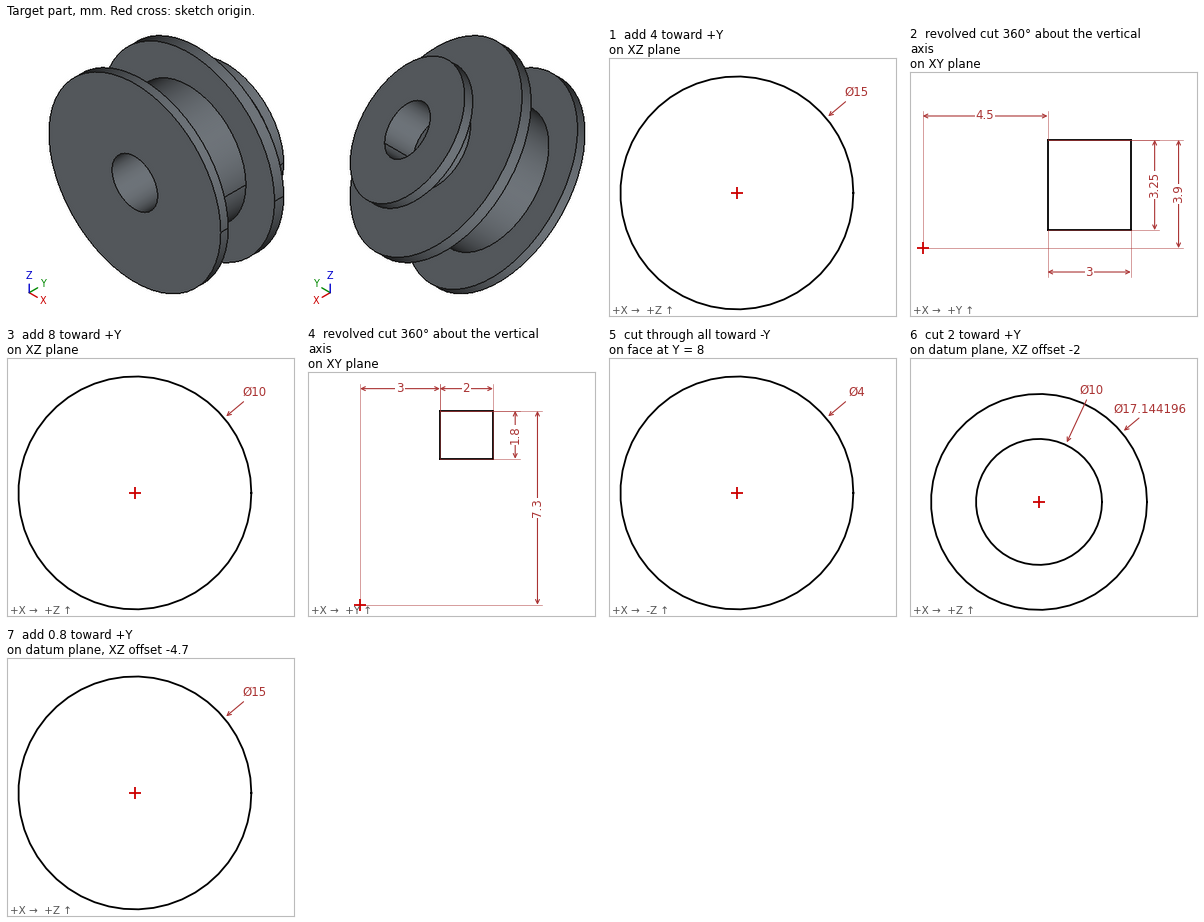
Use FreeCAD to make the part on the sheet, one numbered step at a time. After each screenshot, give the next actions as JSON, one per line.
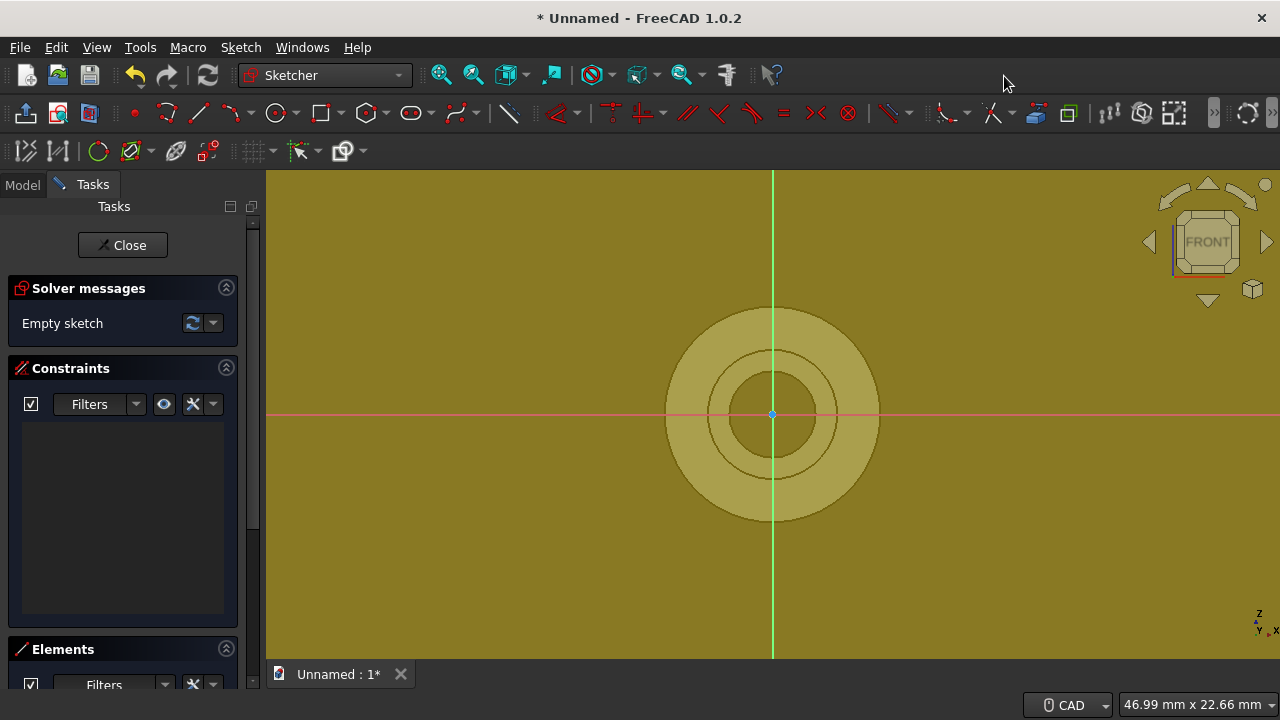
{"action": "key", "text": "g c"}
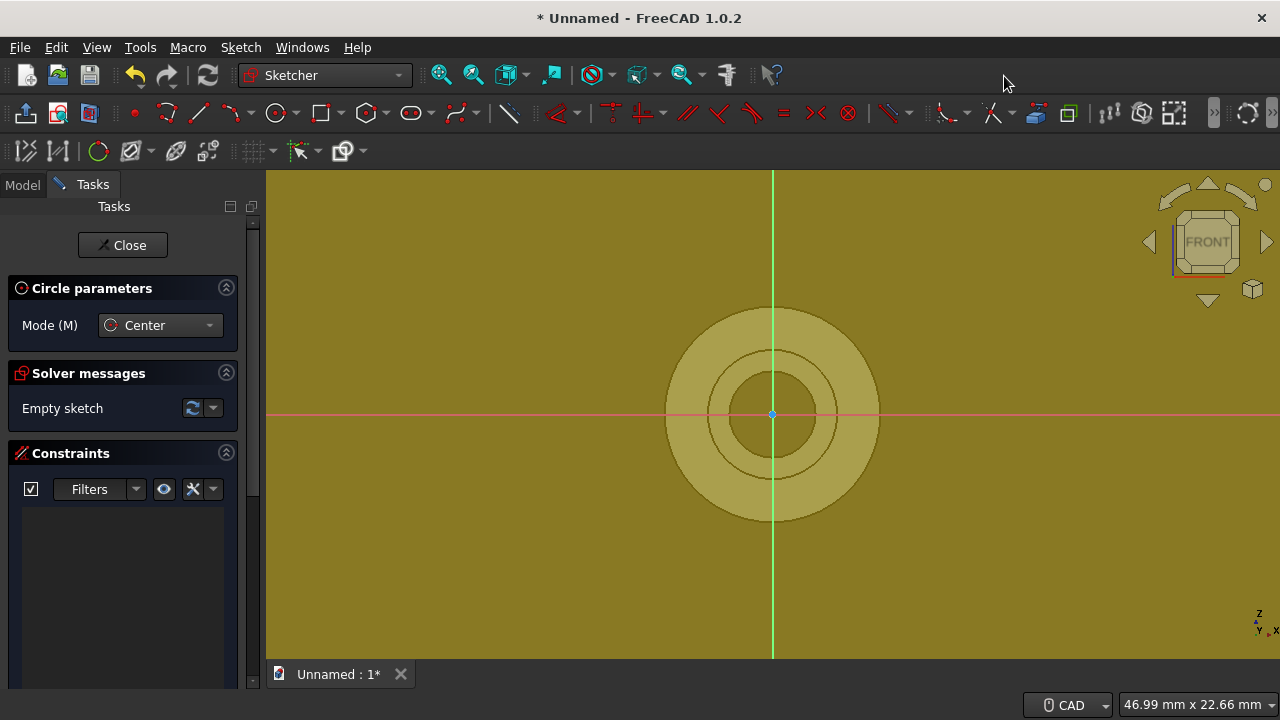
{"action": "left_click", "coordinate": [773, 415]}
{"action": "left_click", "coordinate": [887, 300]}
{"action": "key", "text": "Escape"}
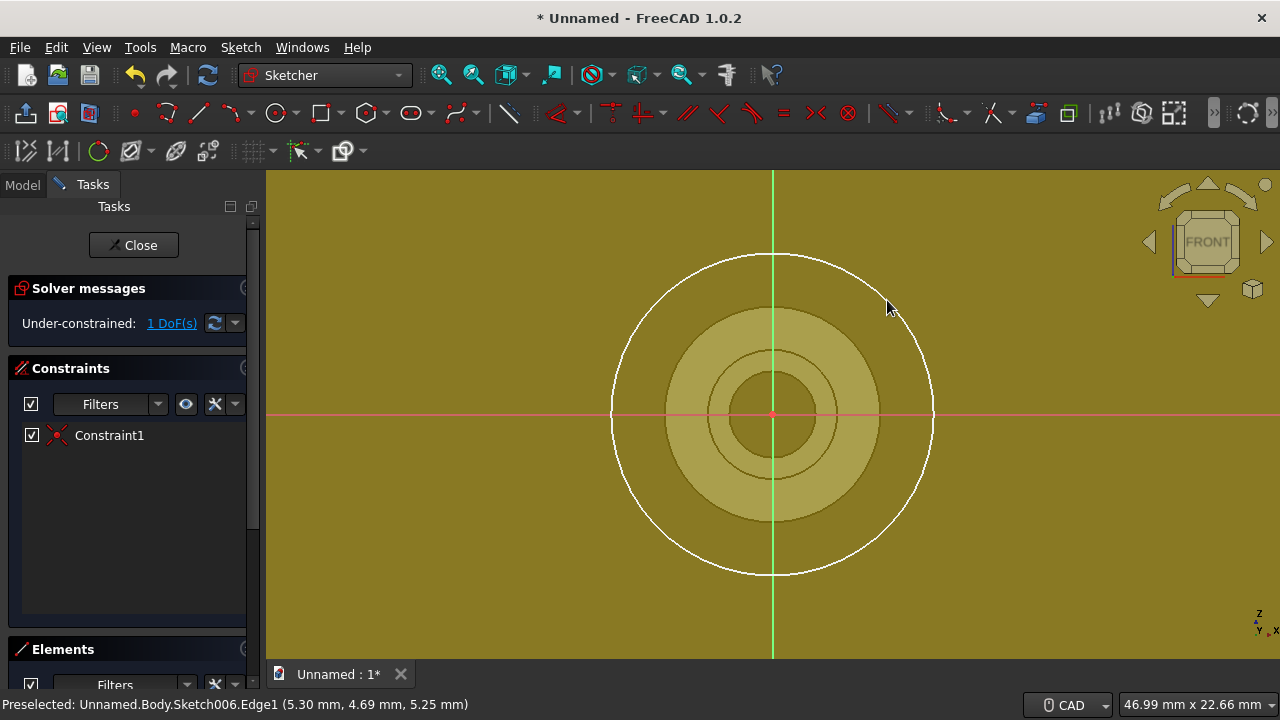
{"action": "key", "text": "d"}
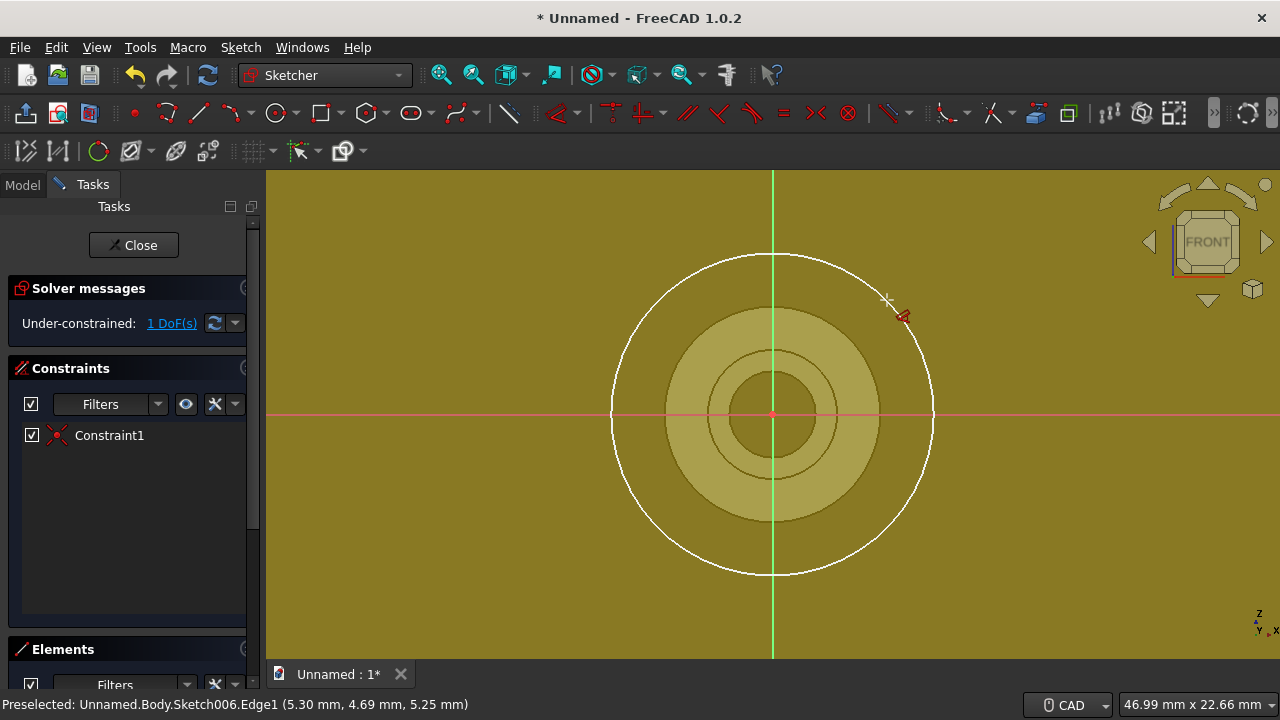
{"action": "left_click", "coordinate": [886, 300]}
{"action": "left_click", "coordinate": [909, 277]}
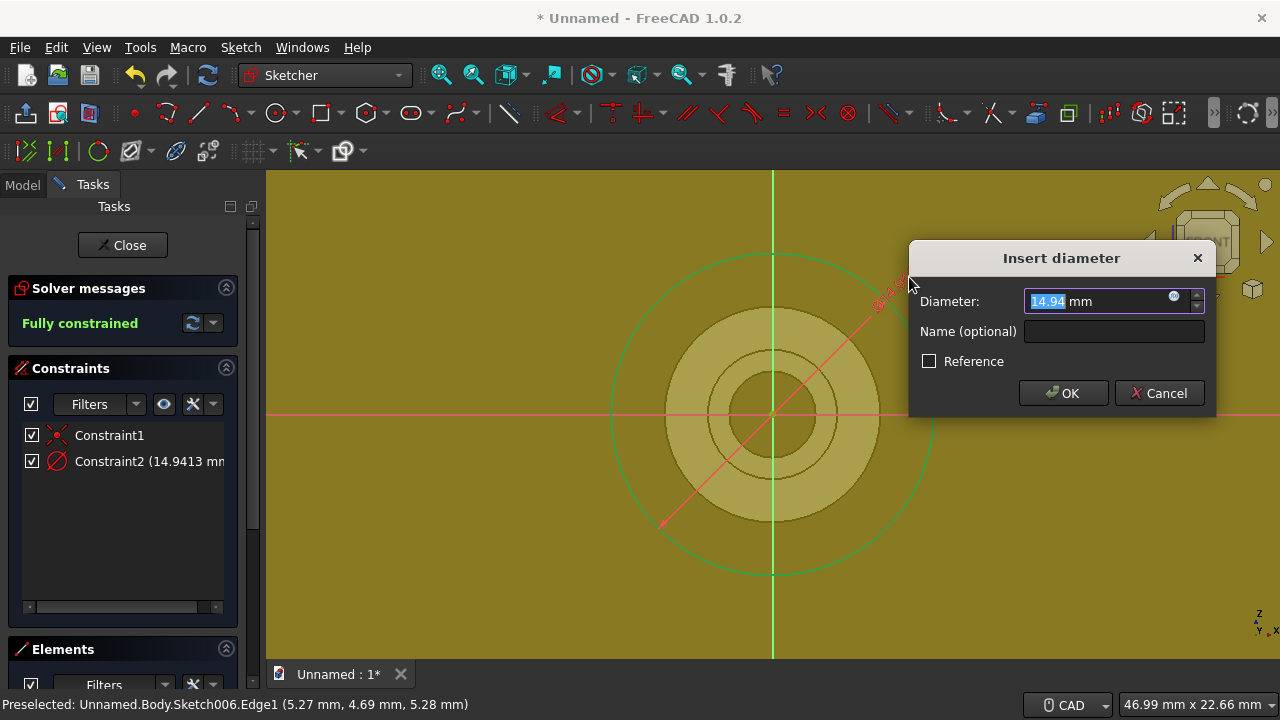
{"action": "type", "text": "15"}
{"action": "key", "text": "Return"}
{"action": "key", "text": "Escape"}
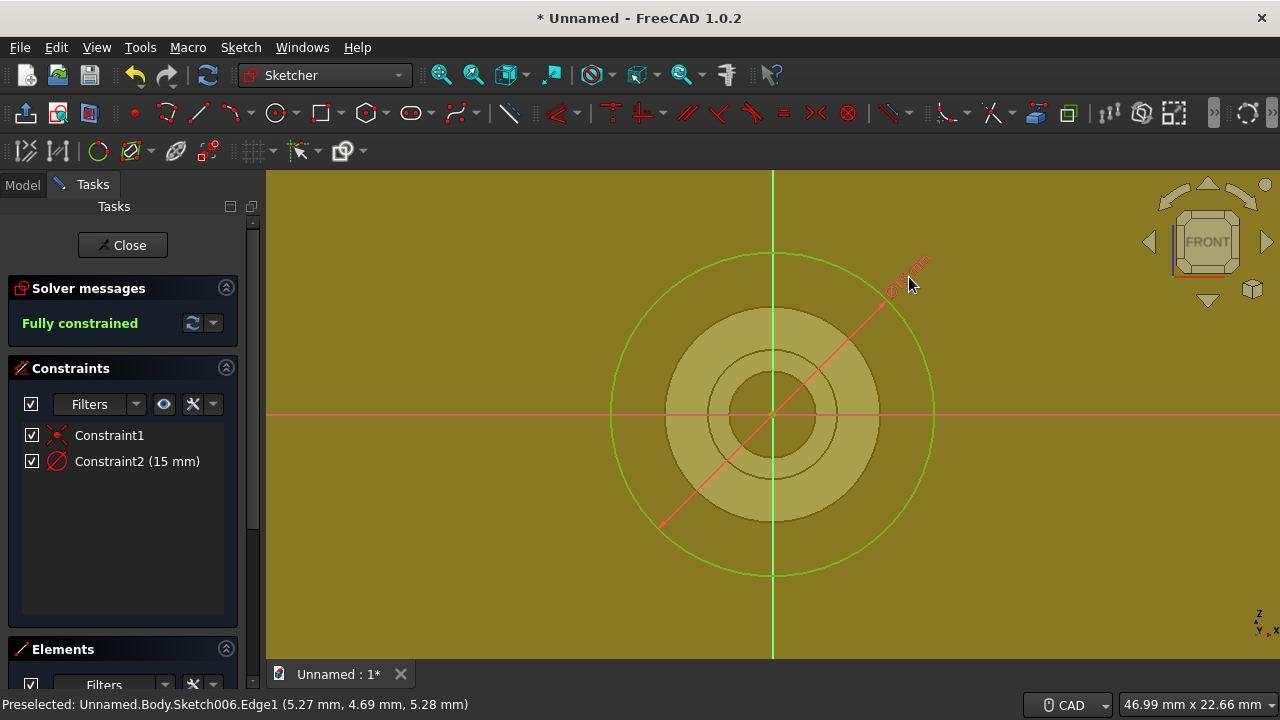
{"action": "left_click", "coordinate": [123, 245]}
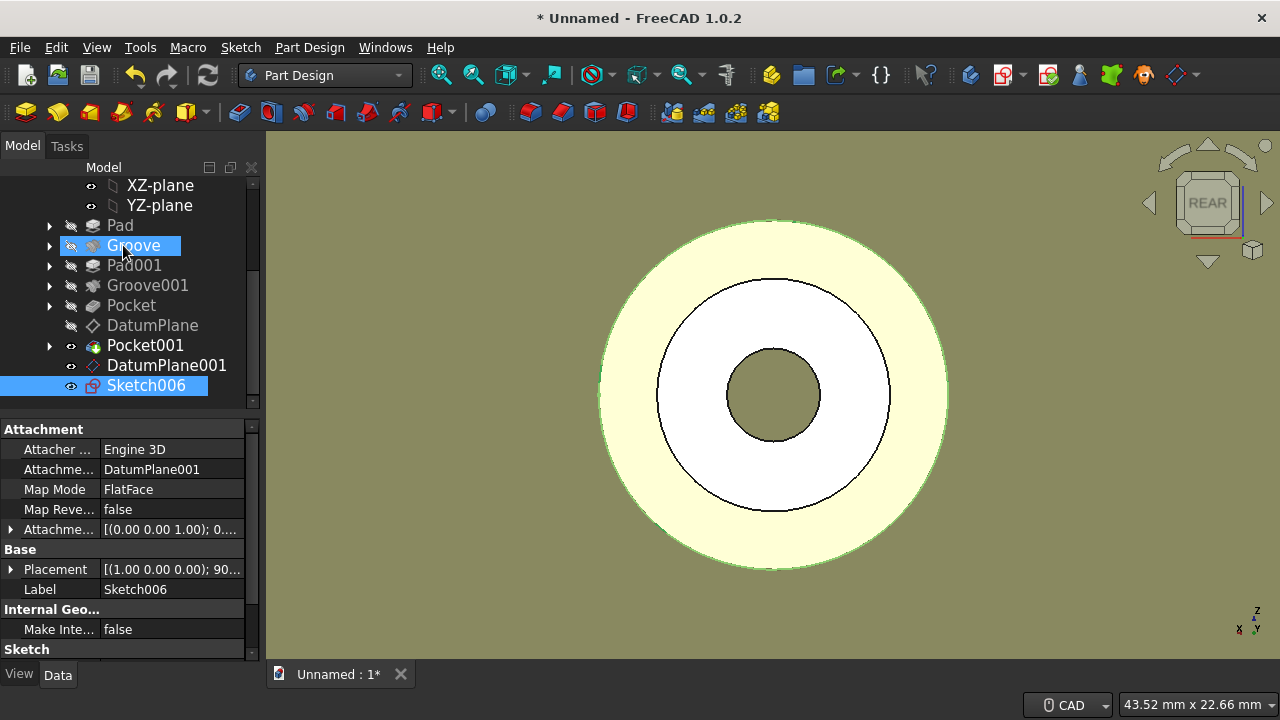
{"action": "left_click", "coordinate": [26, 112]}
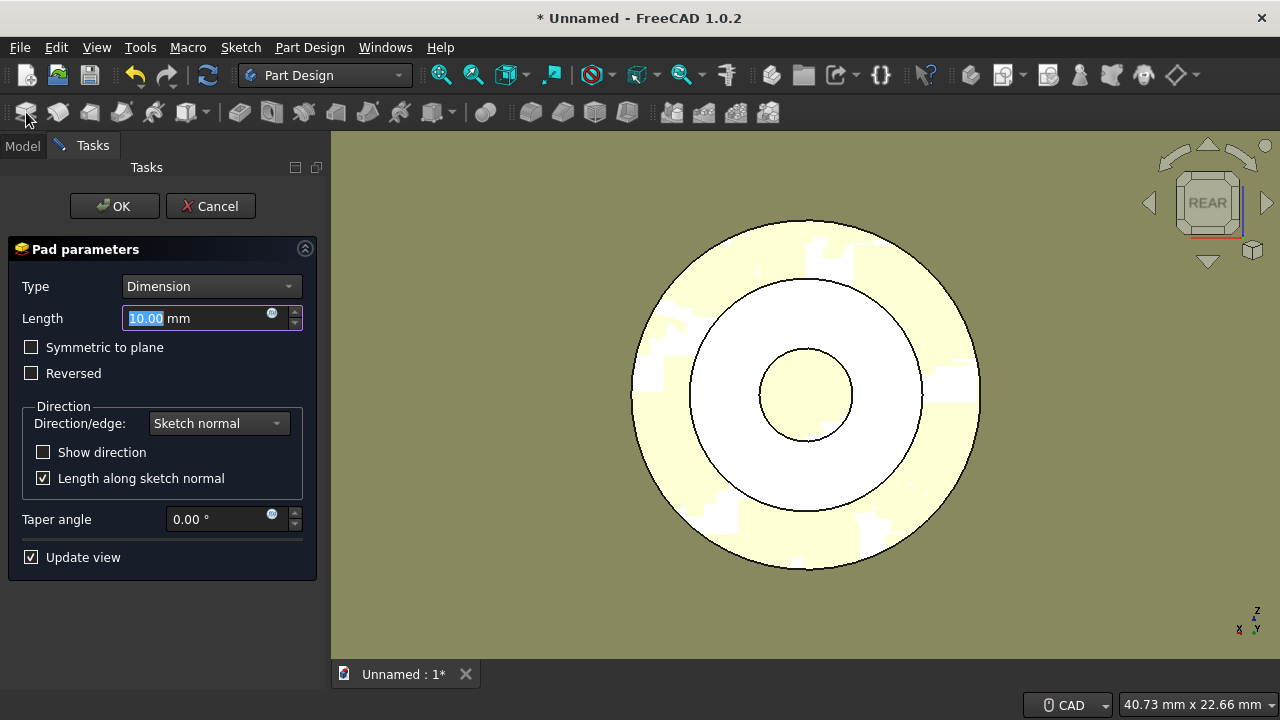
{"action": "type", "text": "0.8"}
{"action": "key", "text": "Tab"}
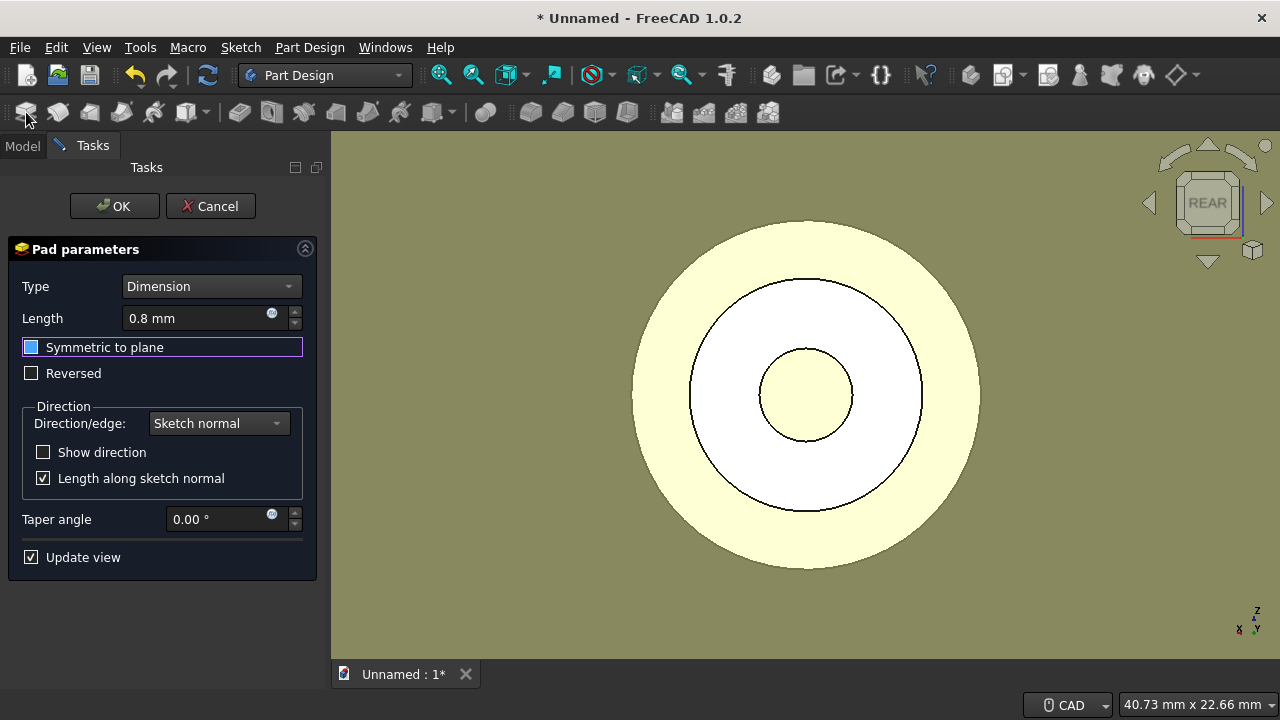
{"action": "left_click", "coordinate": [30, 373]}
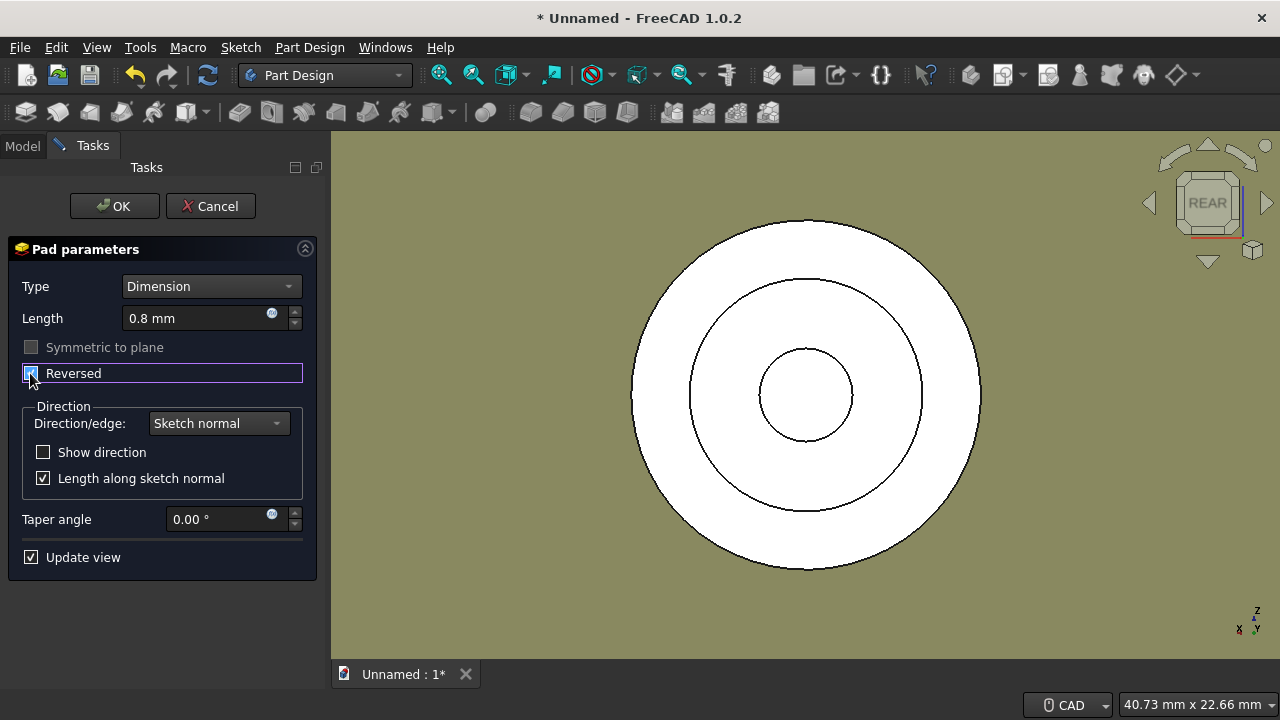
{"action": "left_click", "coordinate": [115, 206]}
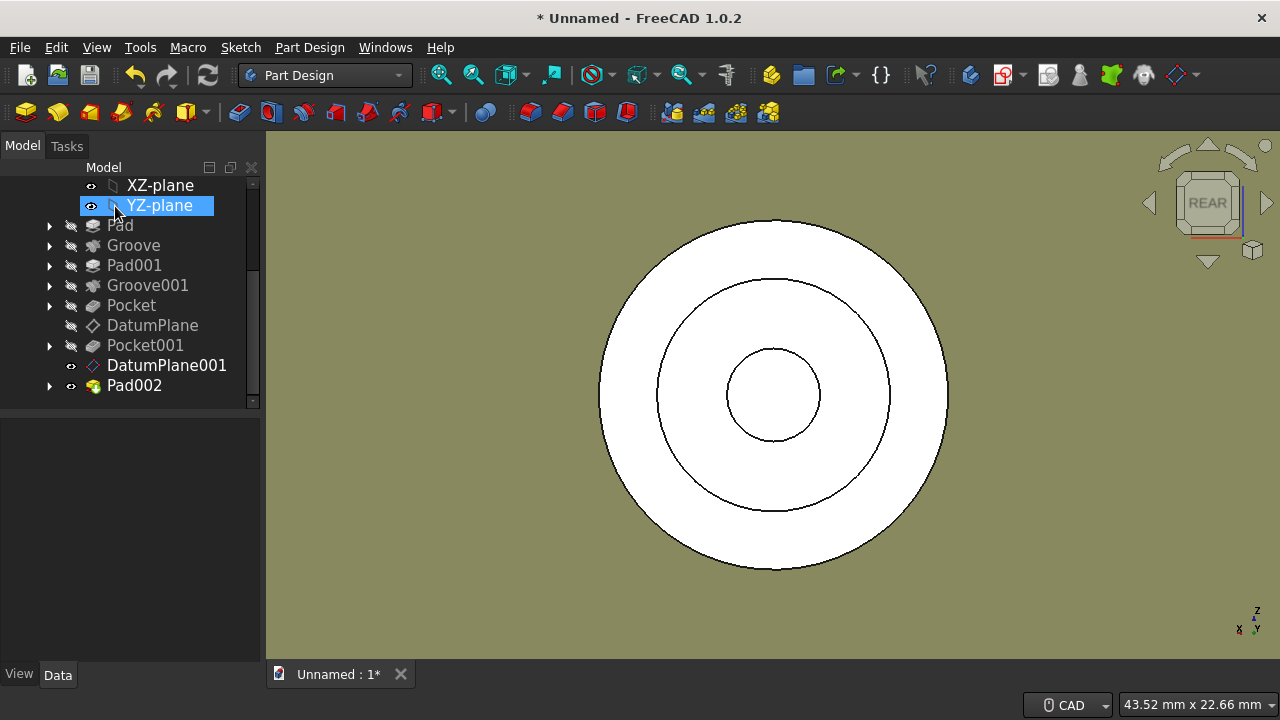
{"action": "left_click", "coordinate": [116, 366]}
{"action": "key", "text": "space"}